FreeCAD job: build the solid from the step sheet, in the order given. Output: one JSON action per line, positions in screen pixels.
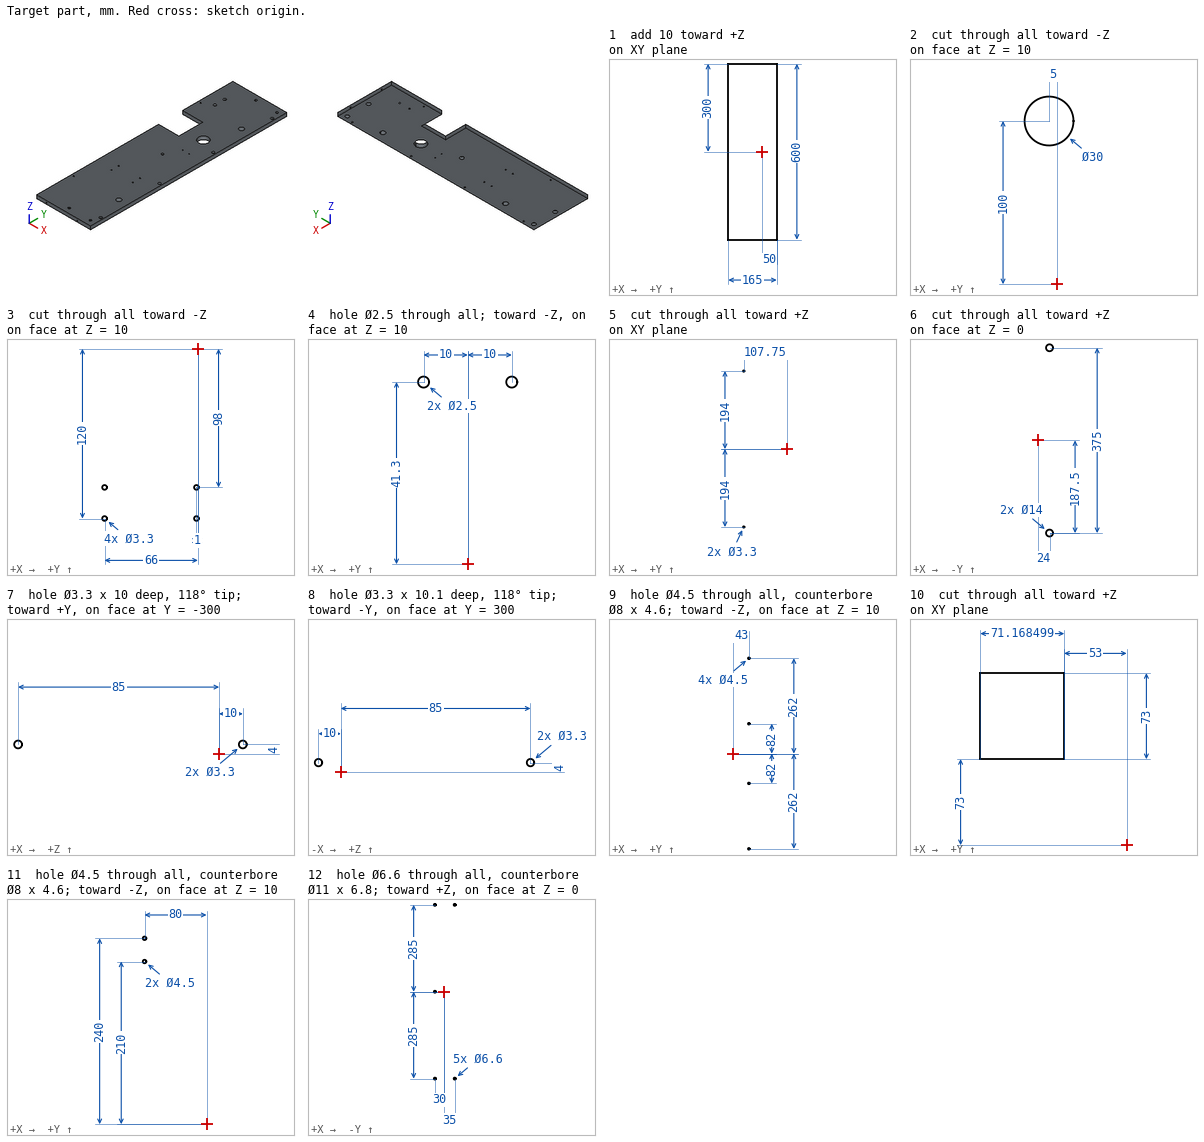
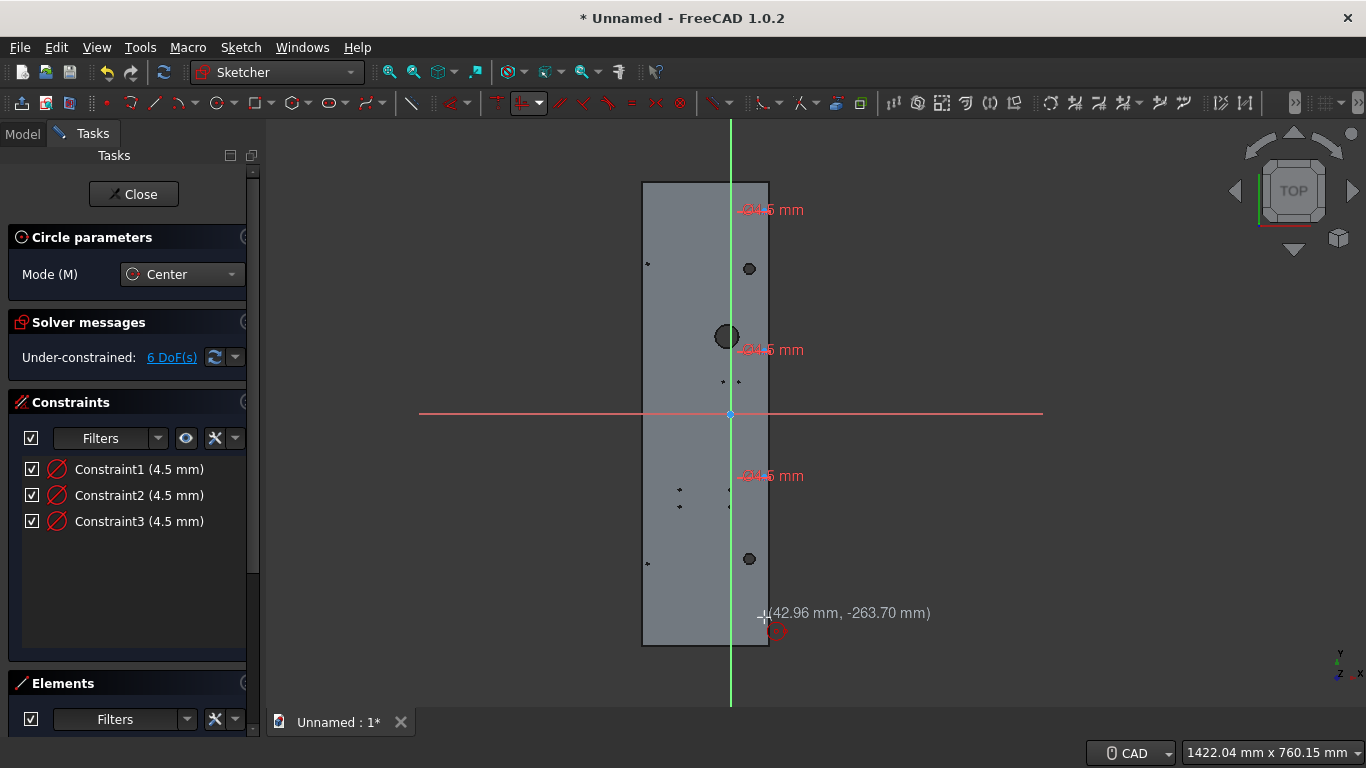
{"action": "left_click", "coordinate": [764, 617]}
{"action": "mouse_move", "coordinate": [765, 615]}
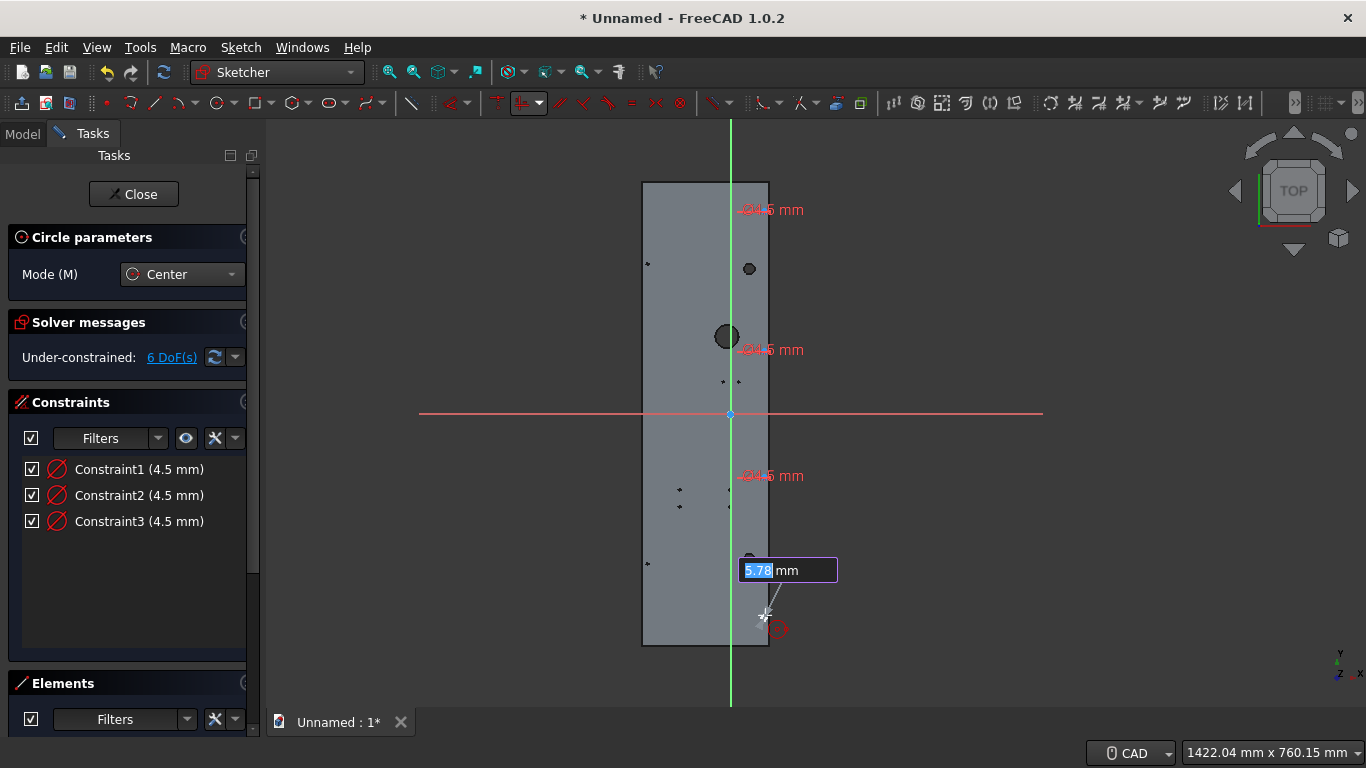
{"action": "type", "text": "4.5"}
{"action": "key", "text": "Return"}
{"action": "key", "text": "Escape"}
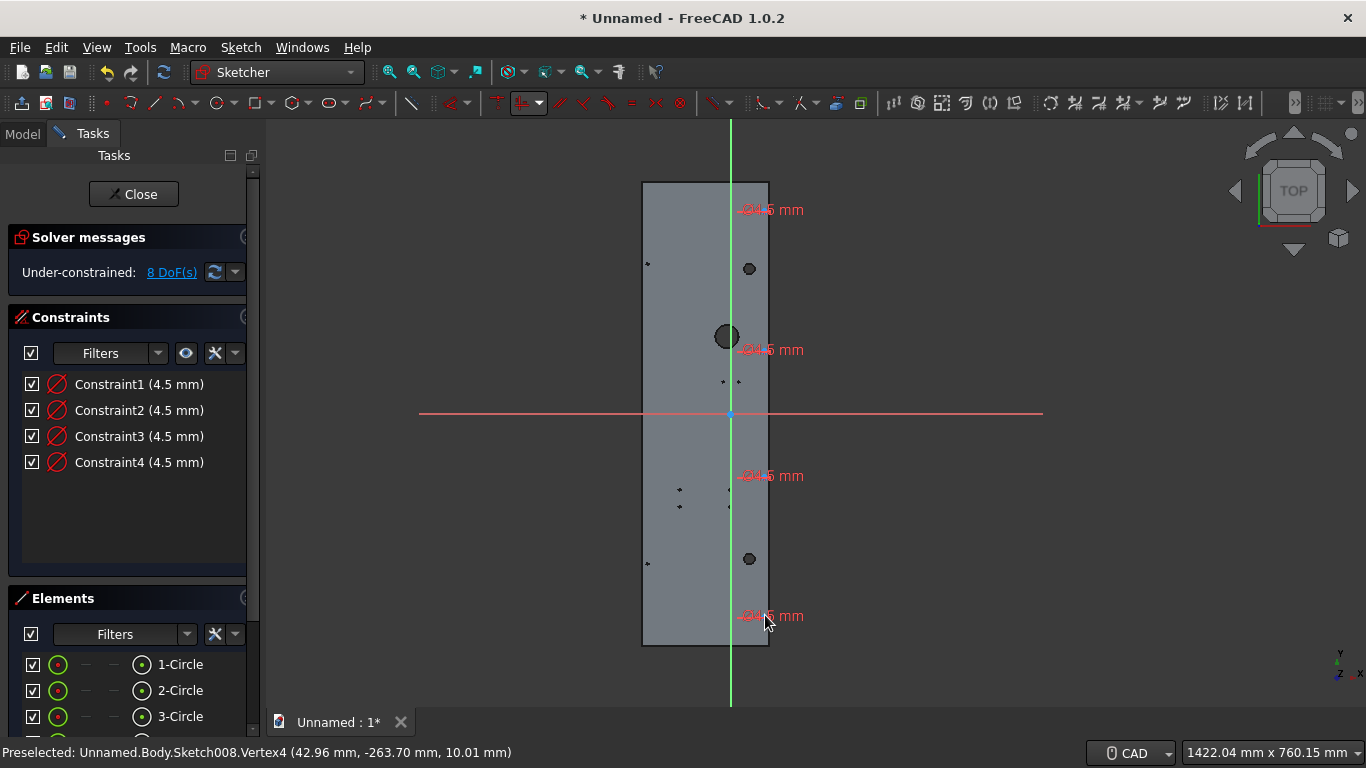
{"action": "left_click", "coordinate": [764, 212]}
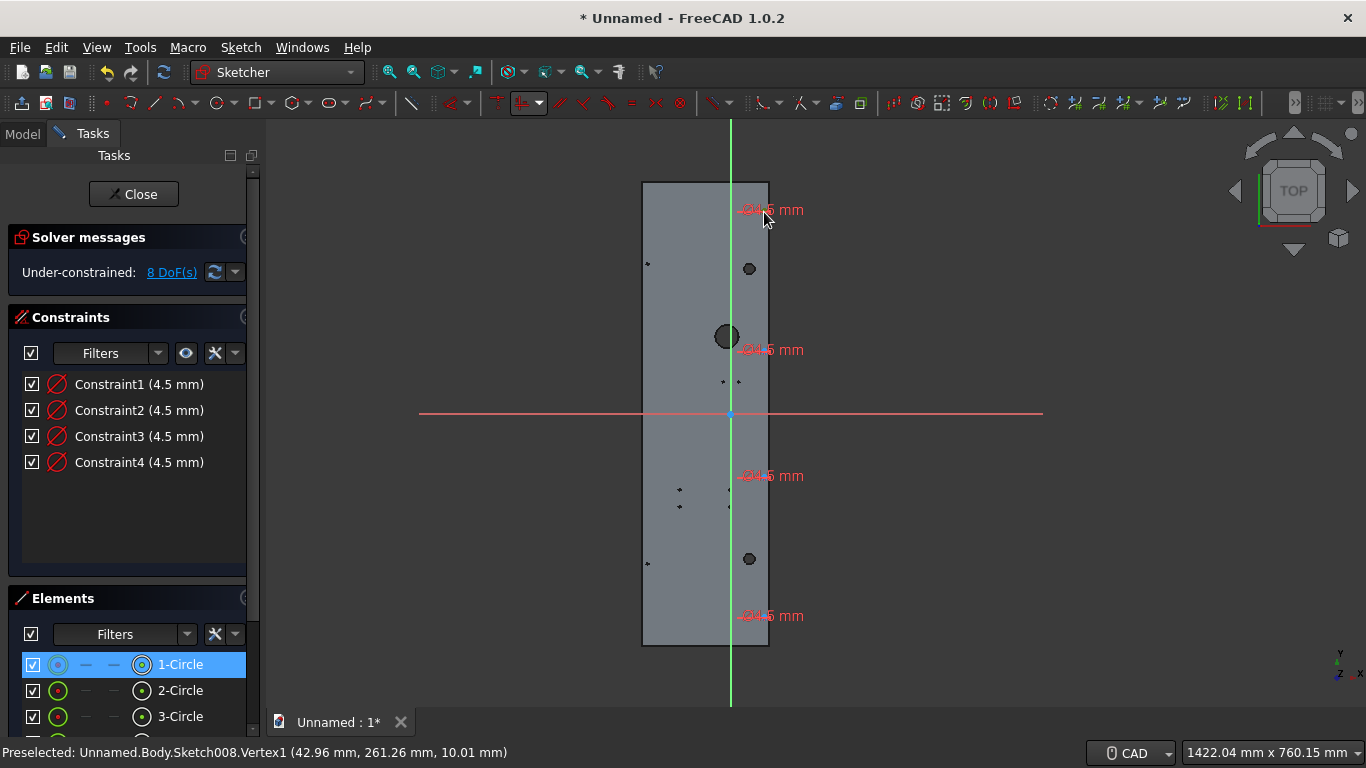
{"action": "left_click", "coordinate": [764, 352]}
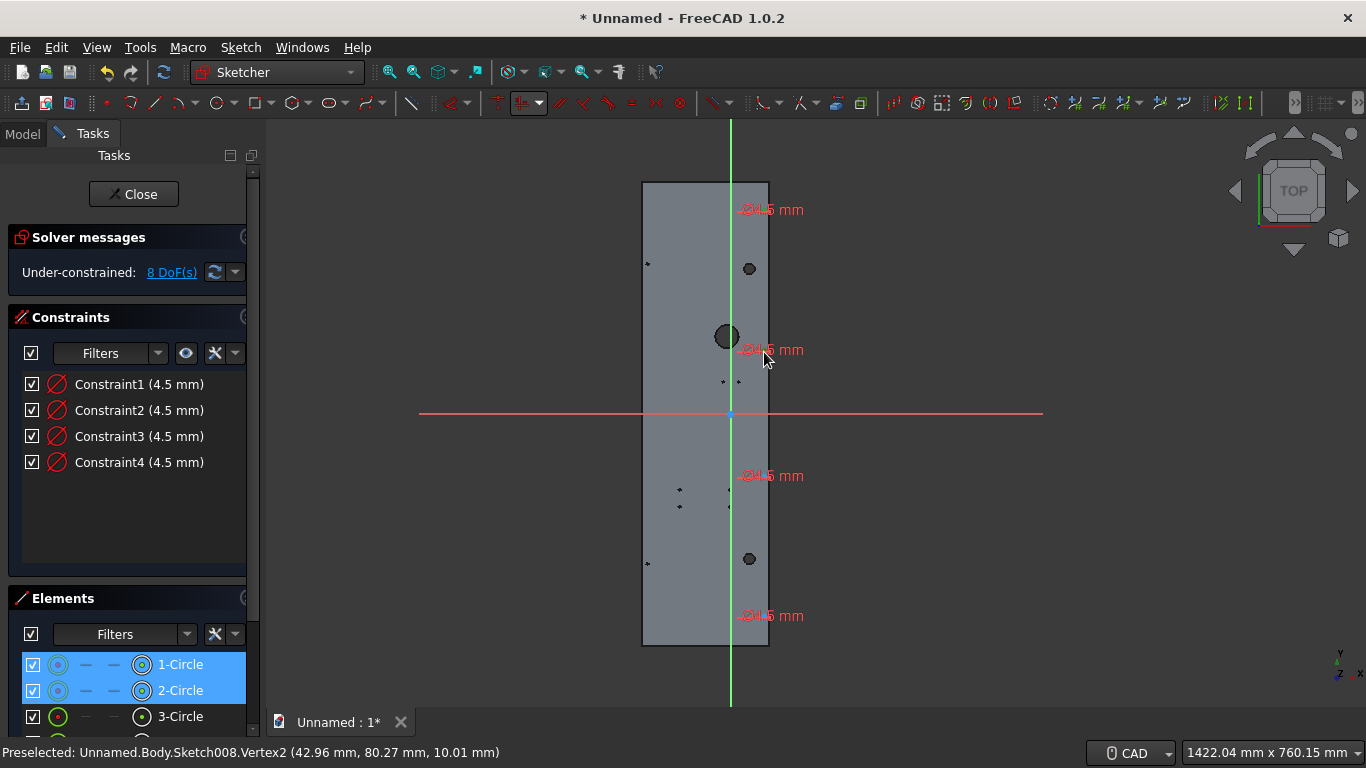
{"action": "key", "text": "v"}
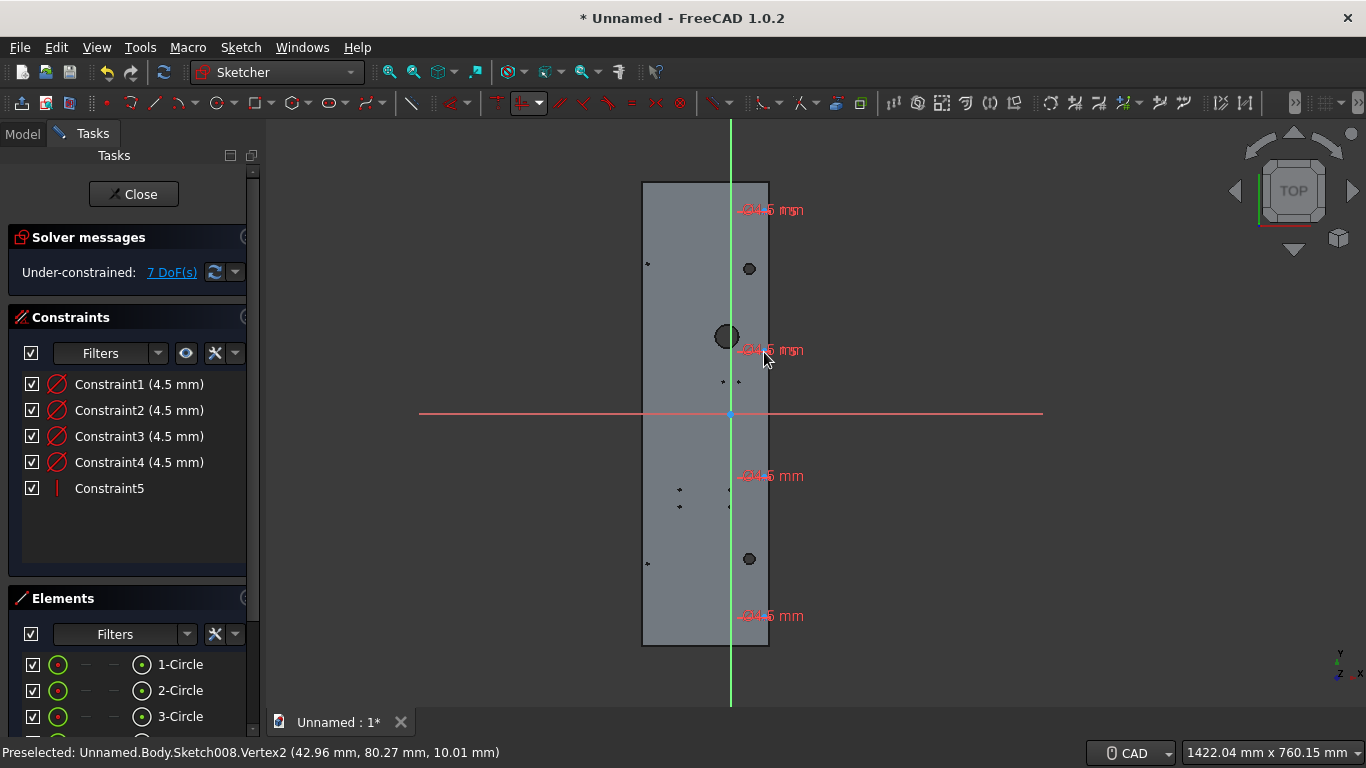
{"action": "left_click", "coordinate": [764, 352]}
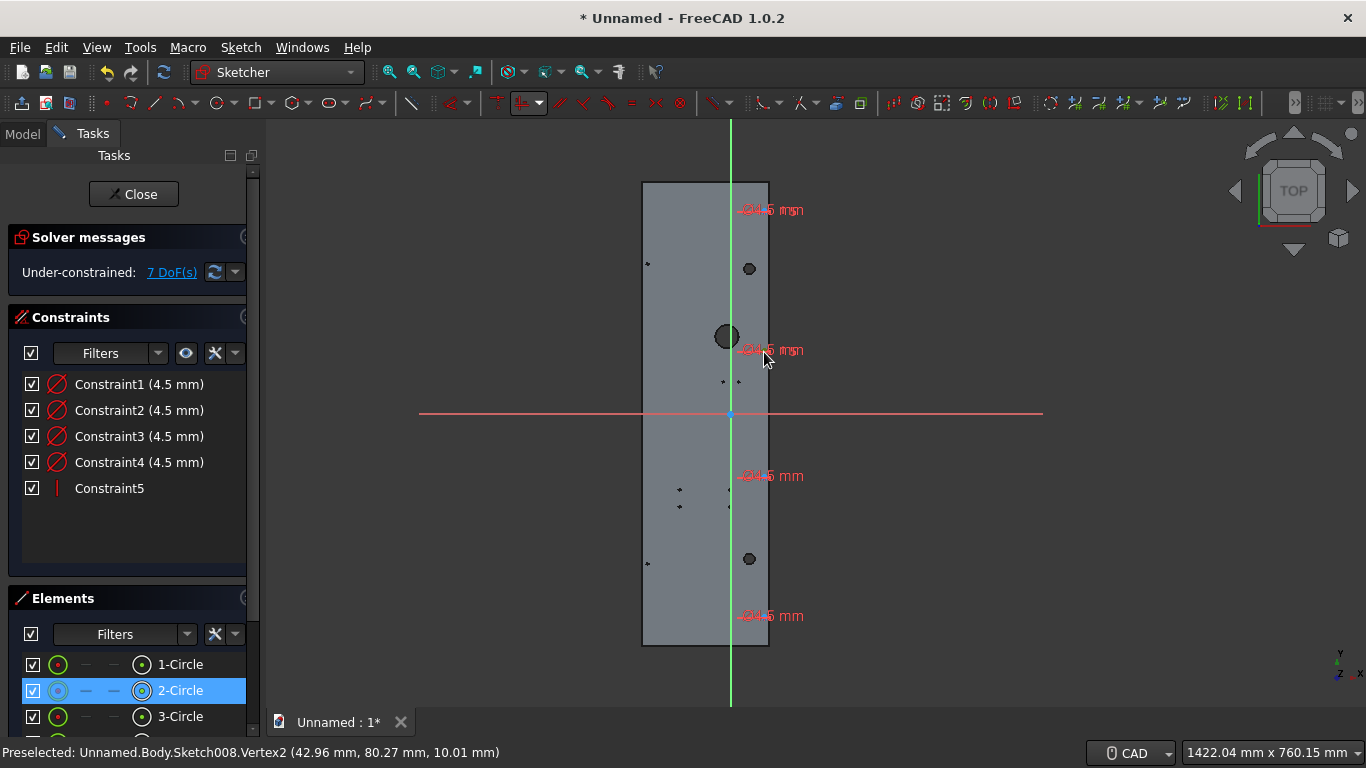
{"action": "left_click", "coordinate": [764, 478]}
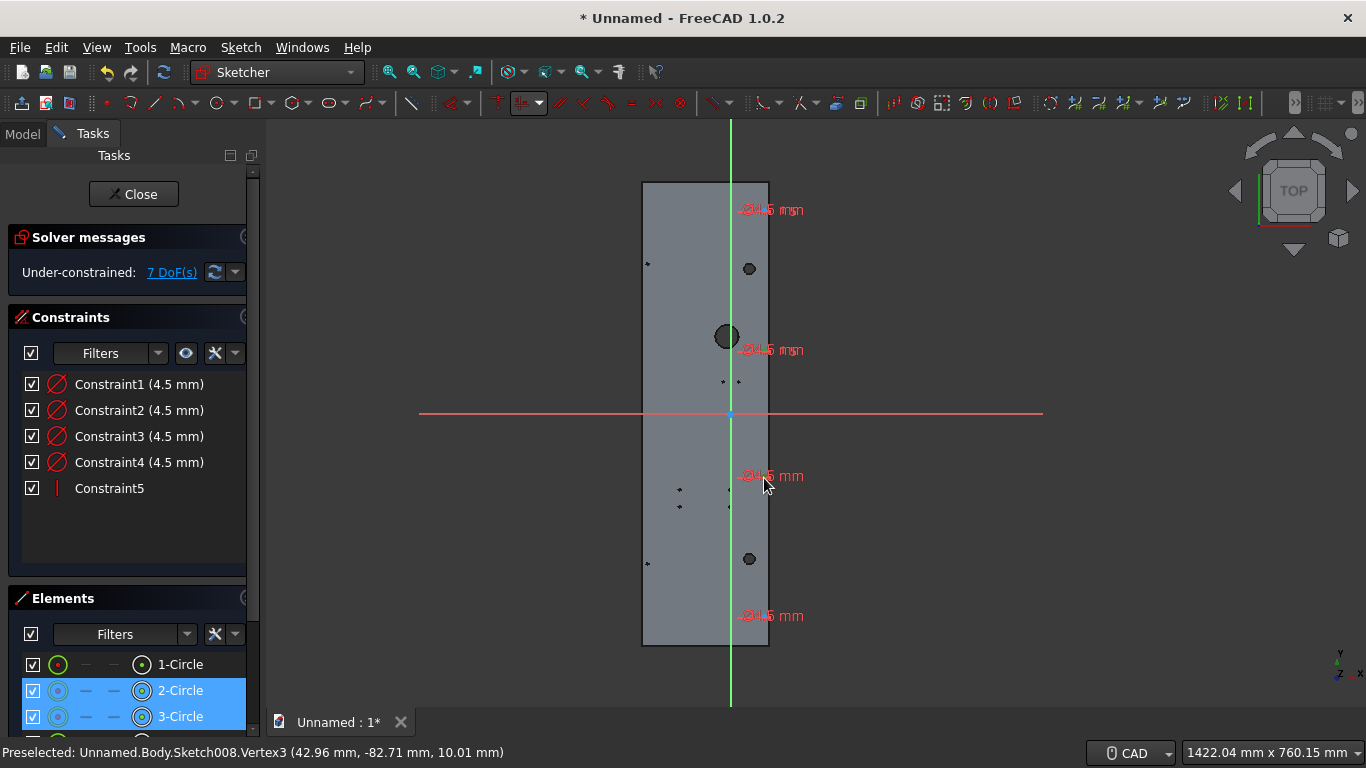
{"action": "left_click", "coordinate": [542, 104]}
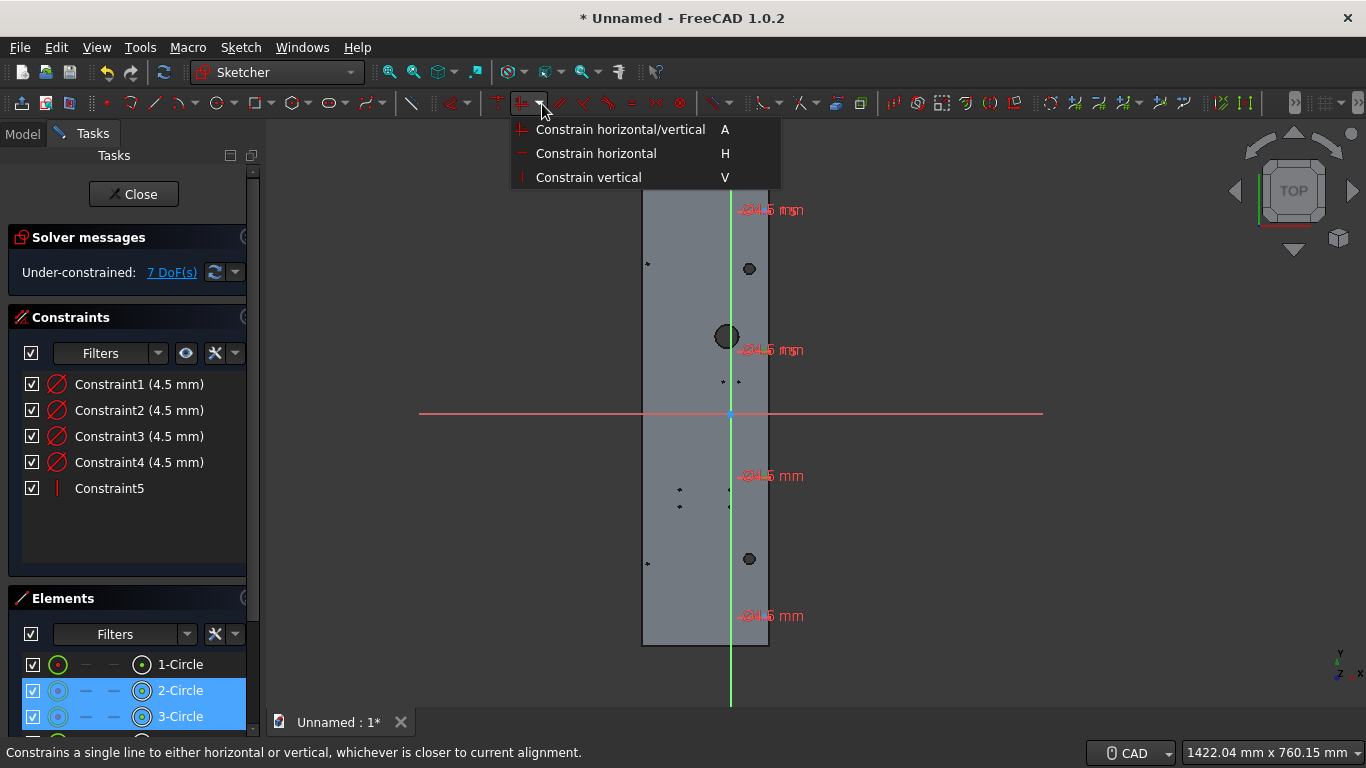
{"action": "left_click", "coordinate": [646, 177]}